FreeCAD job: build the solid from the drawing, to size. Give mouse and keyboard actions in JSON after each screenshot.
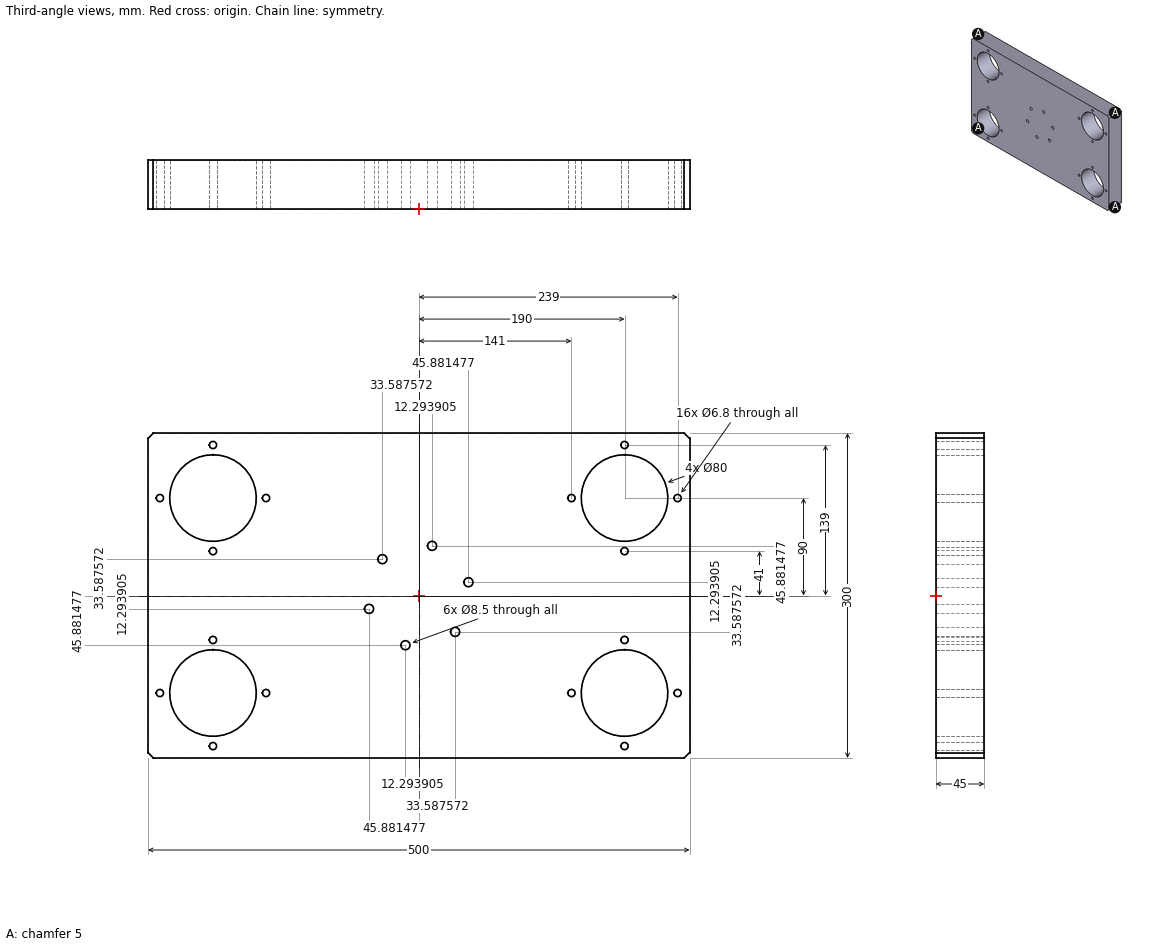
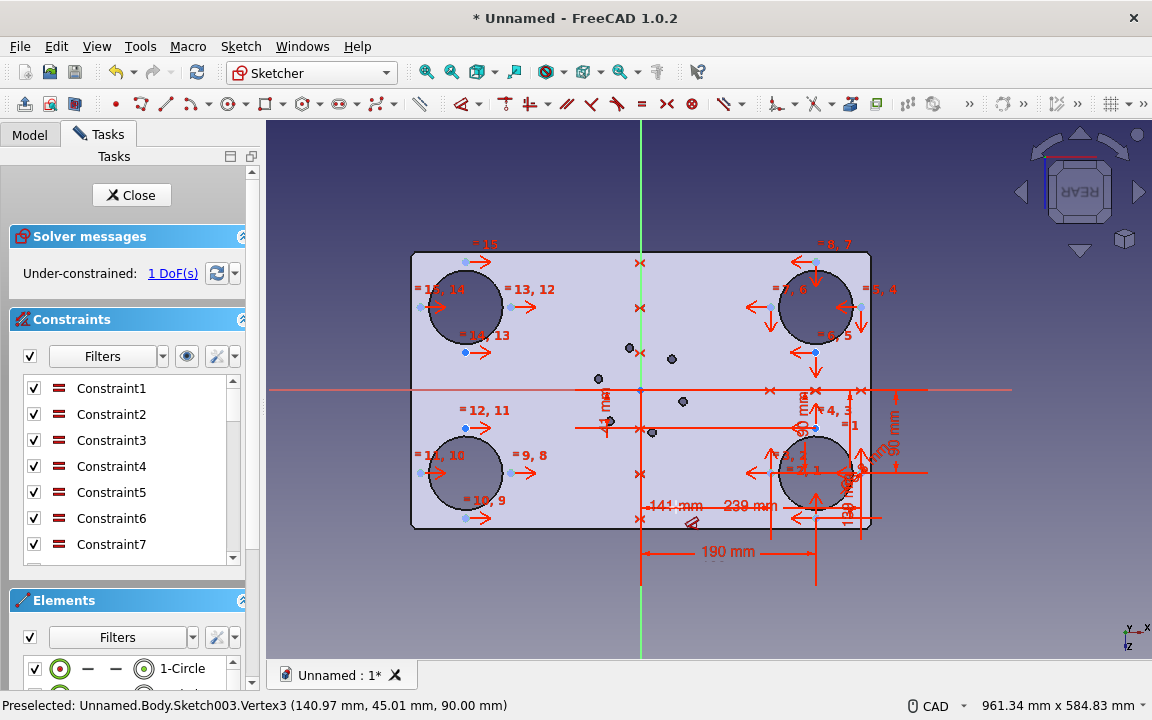
{"action": "left_click", "coordinate": [816, 428]}
{"action": "left_click", "coordinate": [728, 462]}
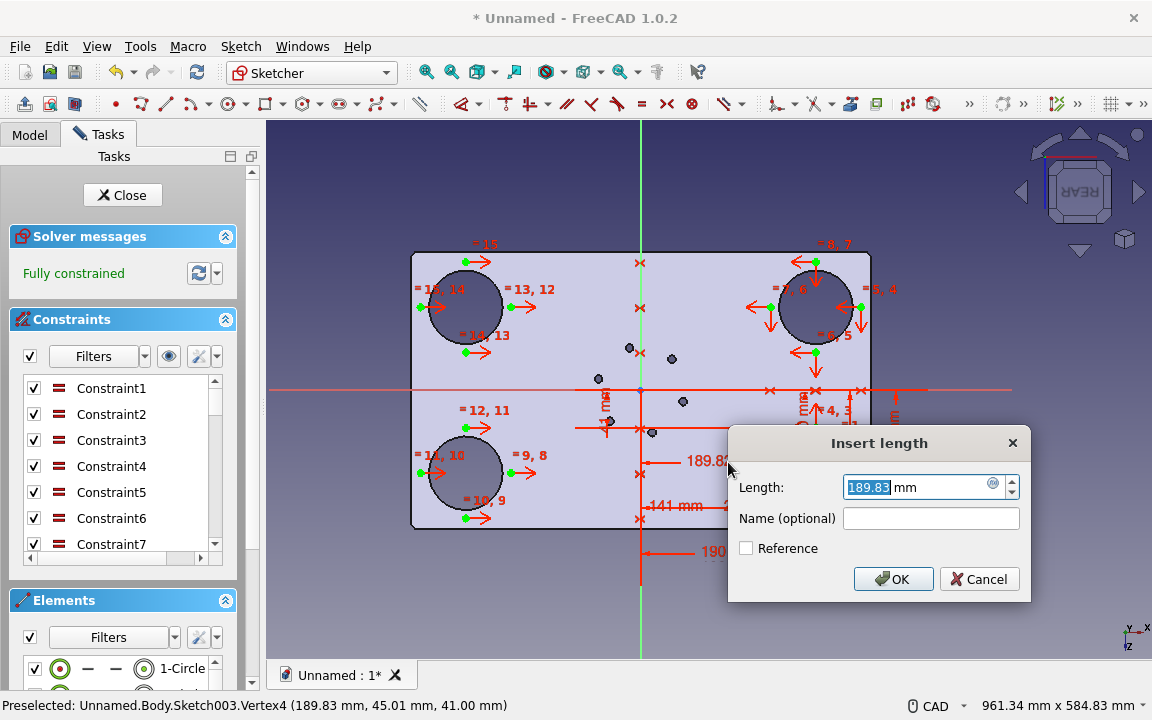
{"action": "type", "text": "190"}
{"action": "key", "text": "Return"}
{"action": "key", "text": "Escape"}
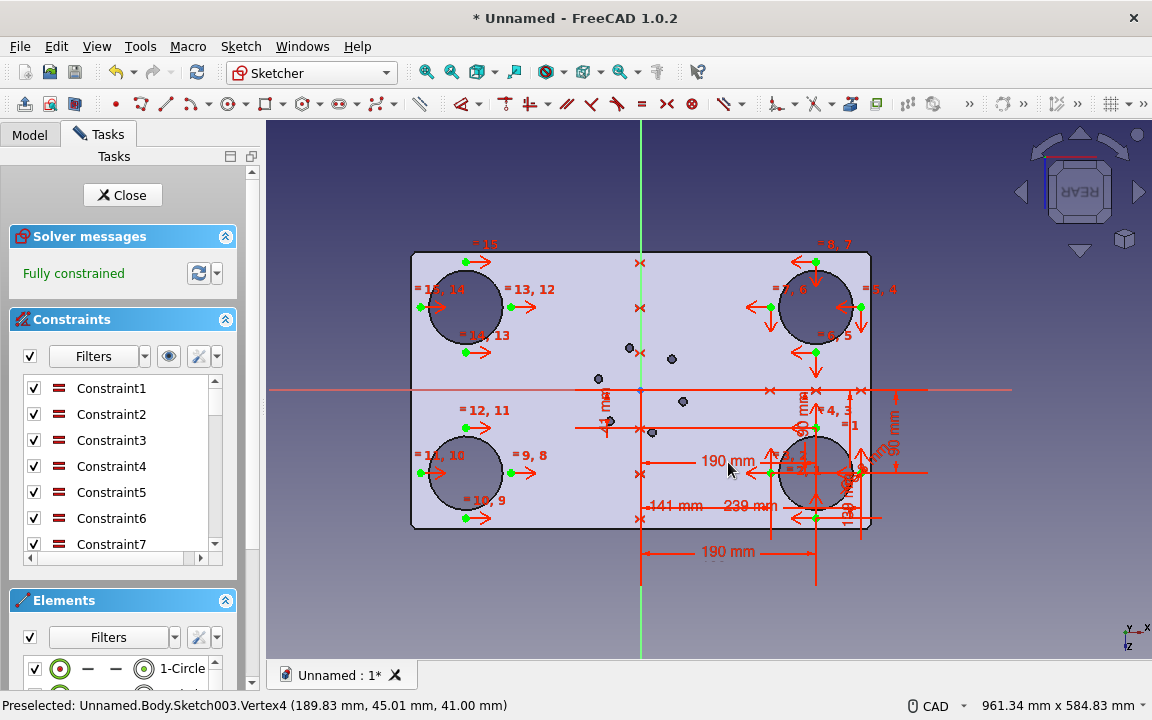
{"action": "left_click", "coordinate": [123, 195]}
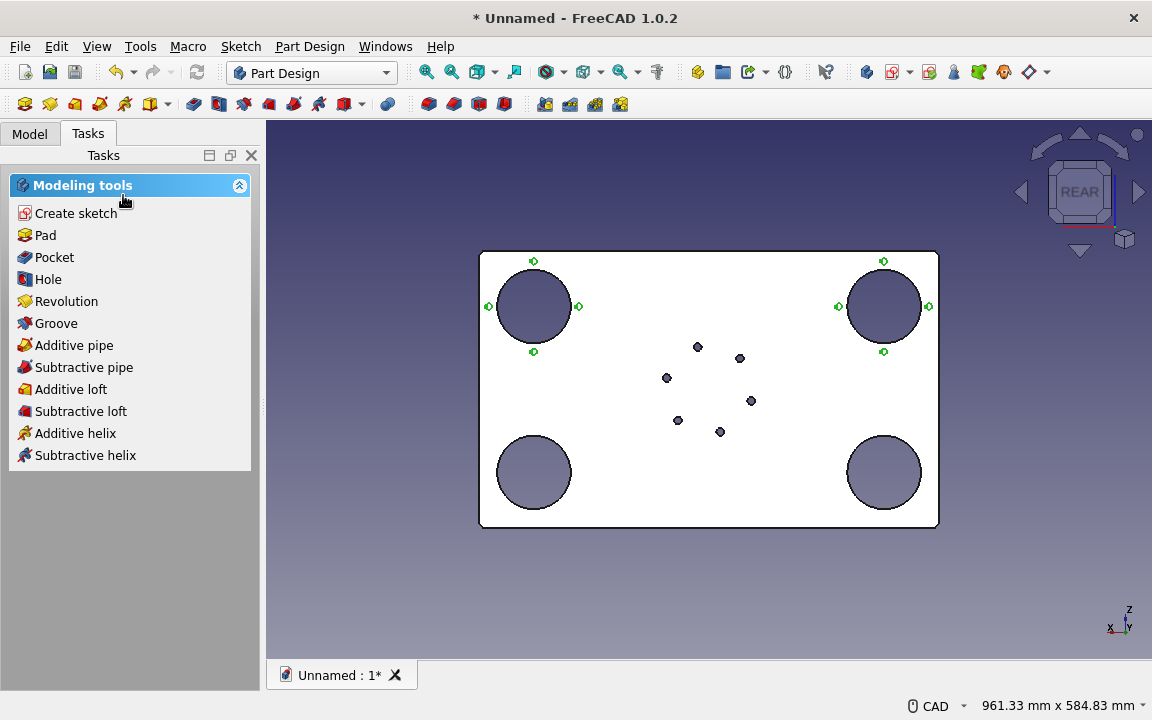
{"action": "left_click", "coordinate": [219, 104]}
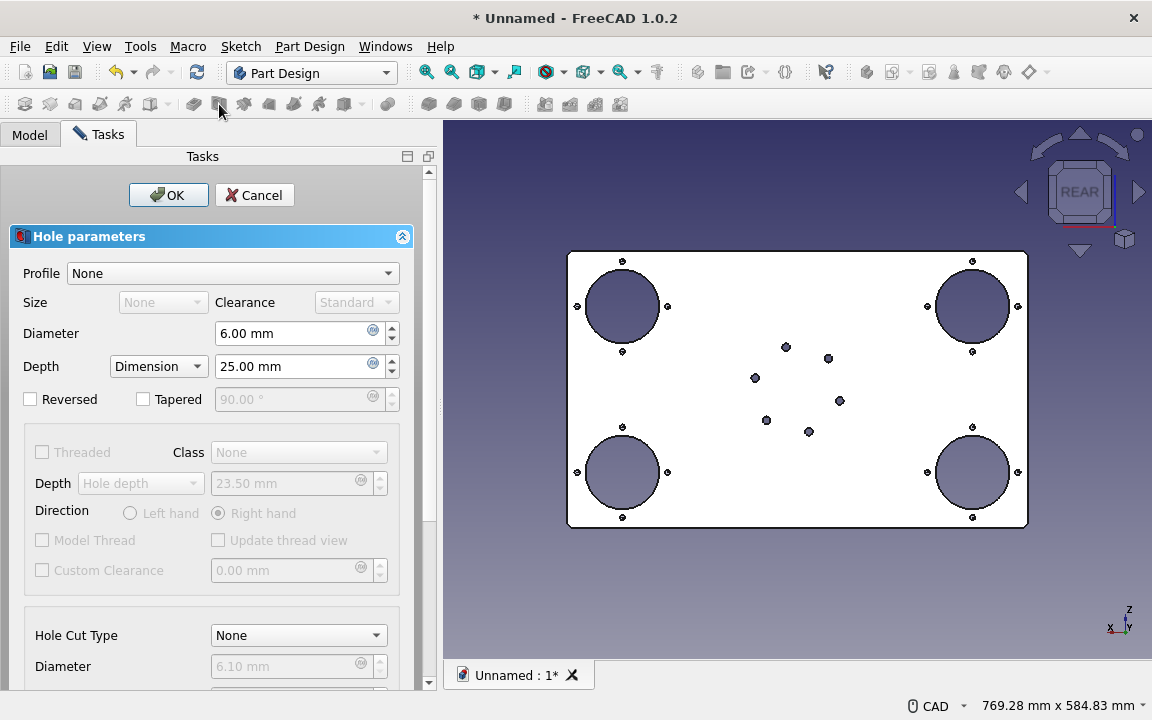
{"action": "triple_click", "coordinate": [300, 334]}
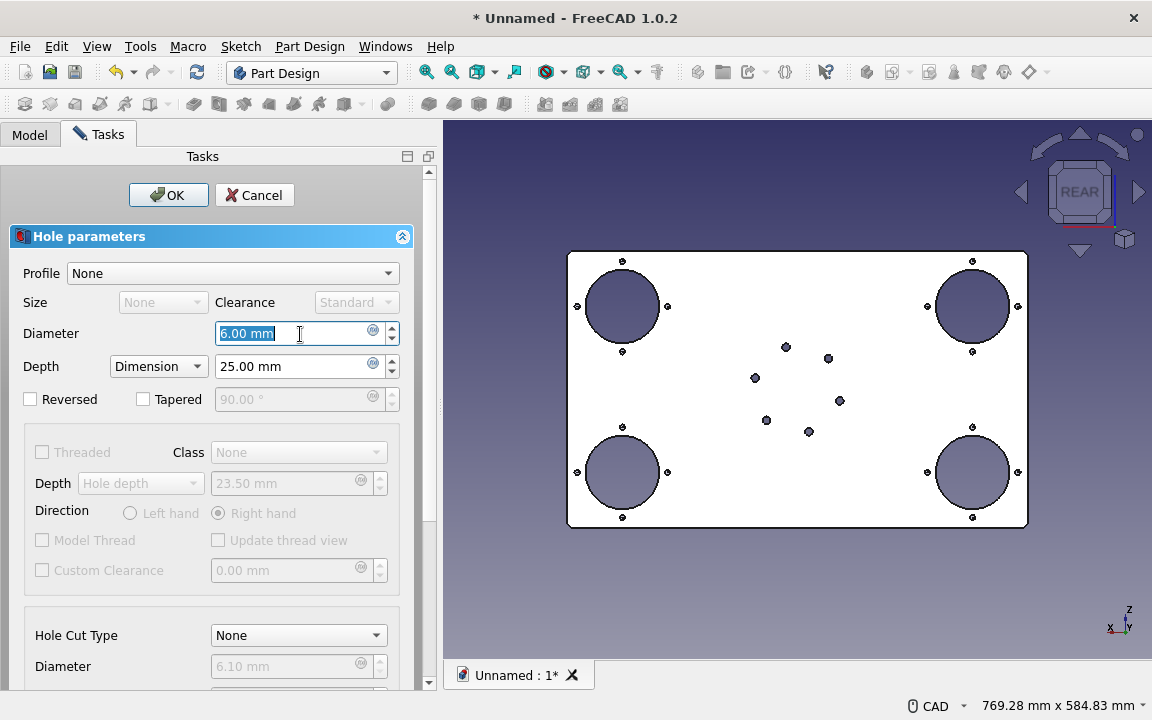
{"action": "type", "text": "6.8"}
{"action": "key", "text": "Tab"}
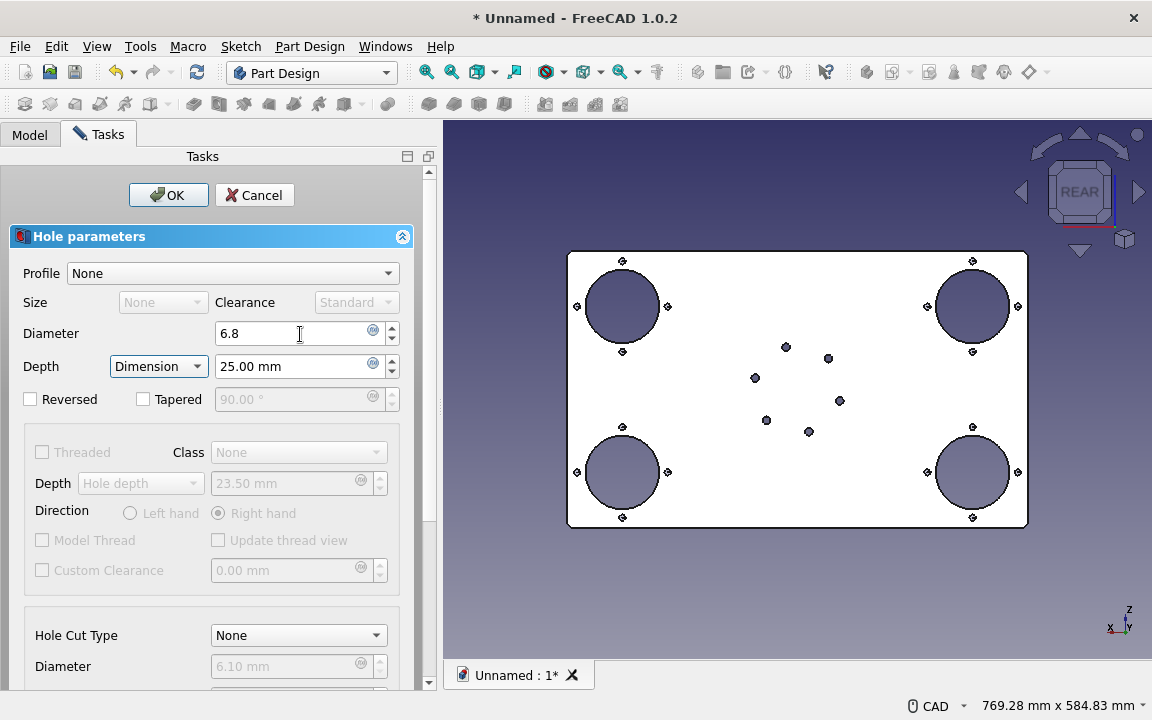
{"action": "left_click", "coordinate": [160, 366]}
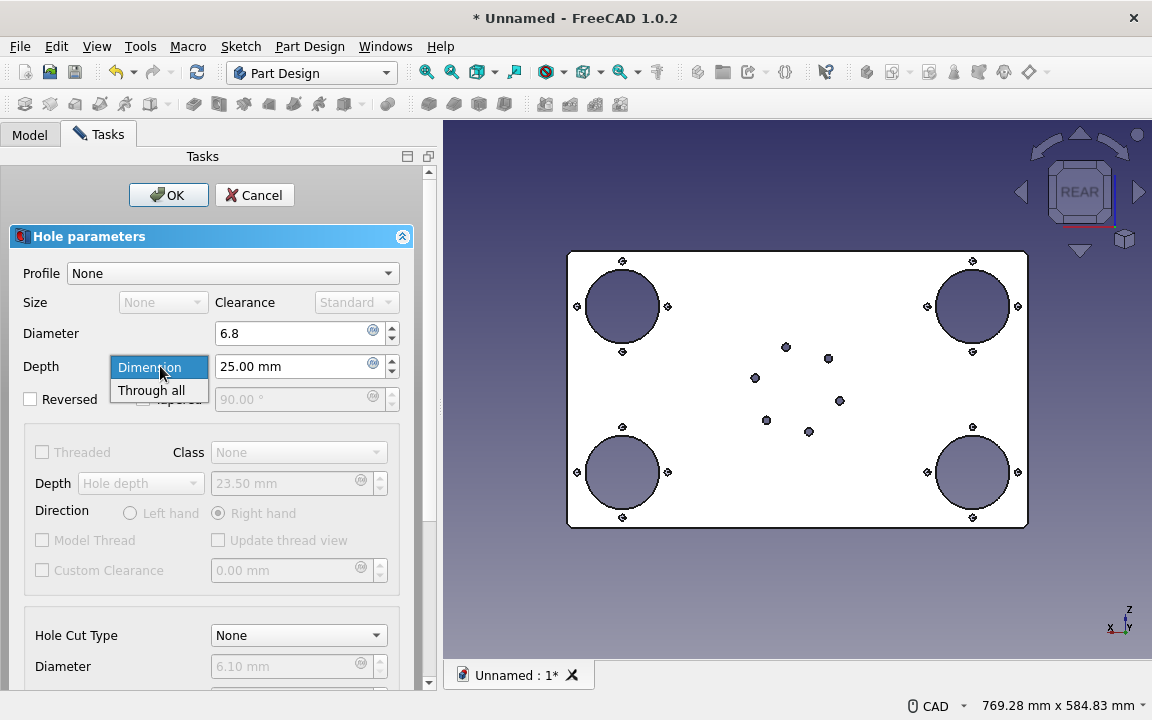
{"action": "left_click", "coordinate": [158, 390]}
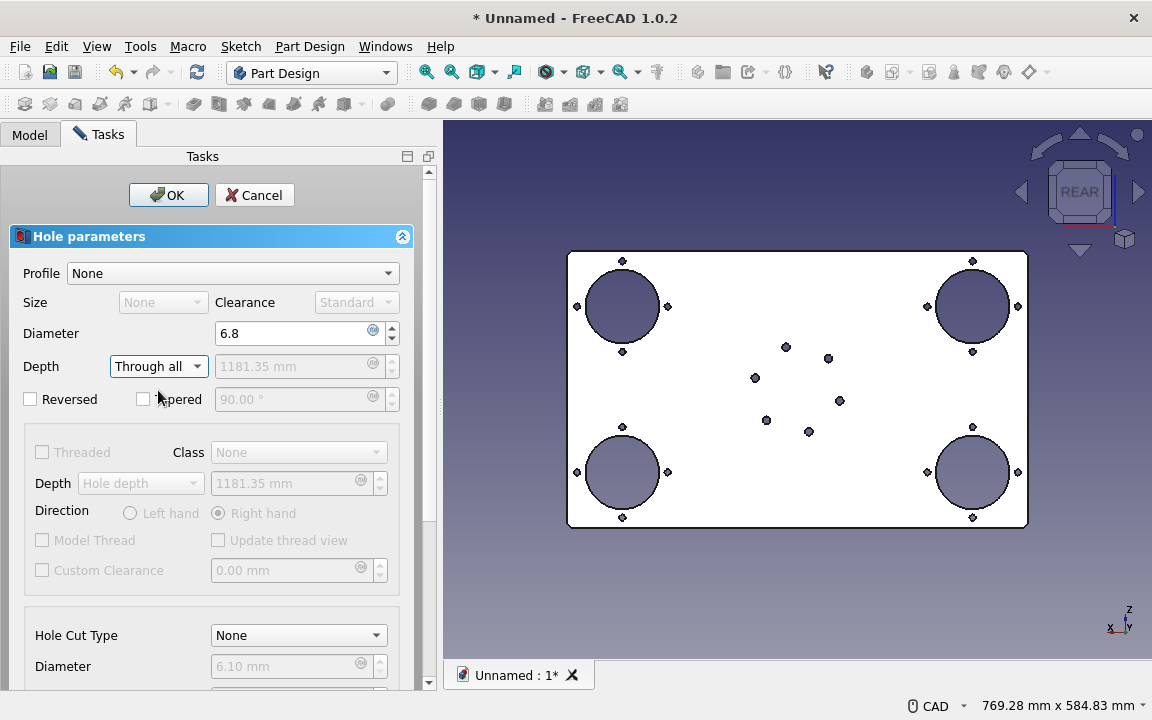
{"action": "left_click", "coordinate": [169, 195]}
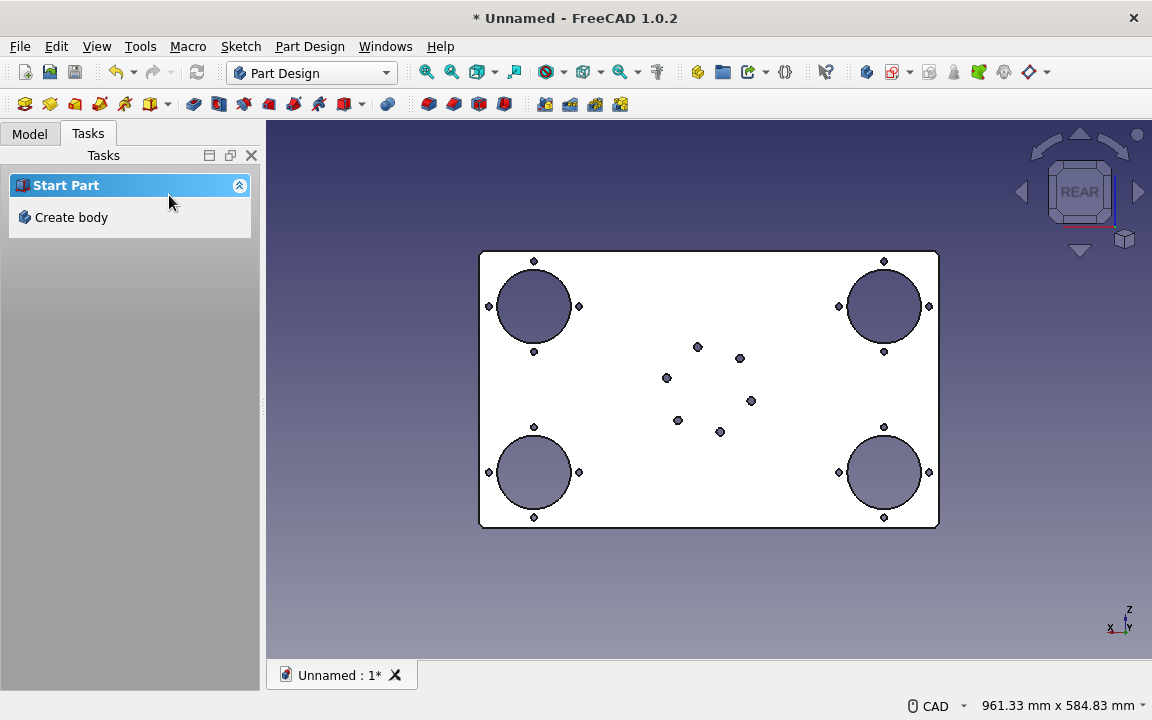
{"action": "key", "text": "0"}